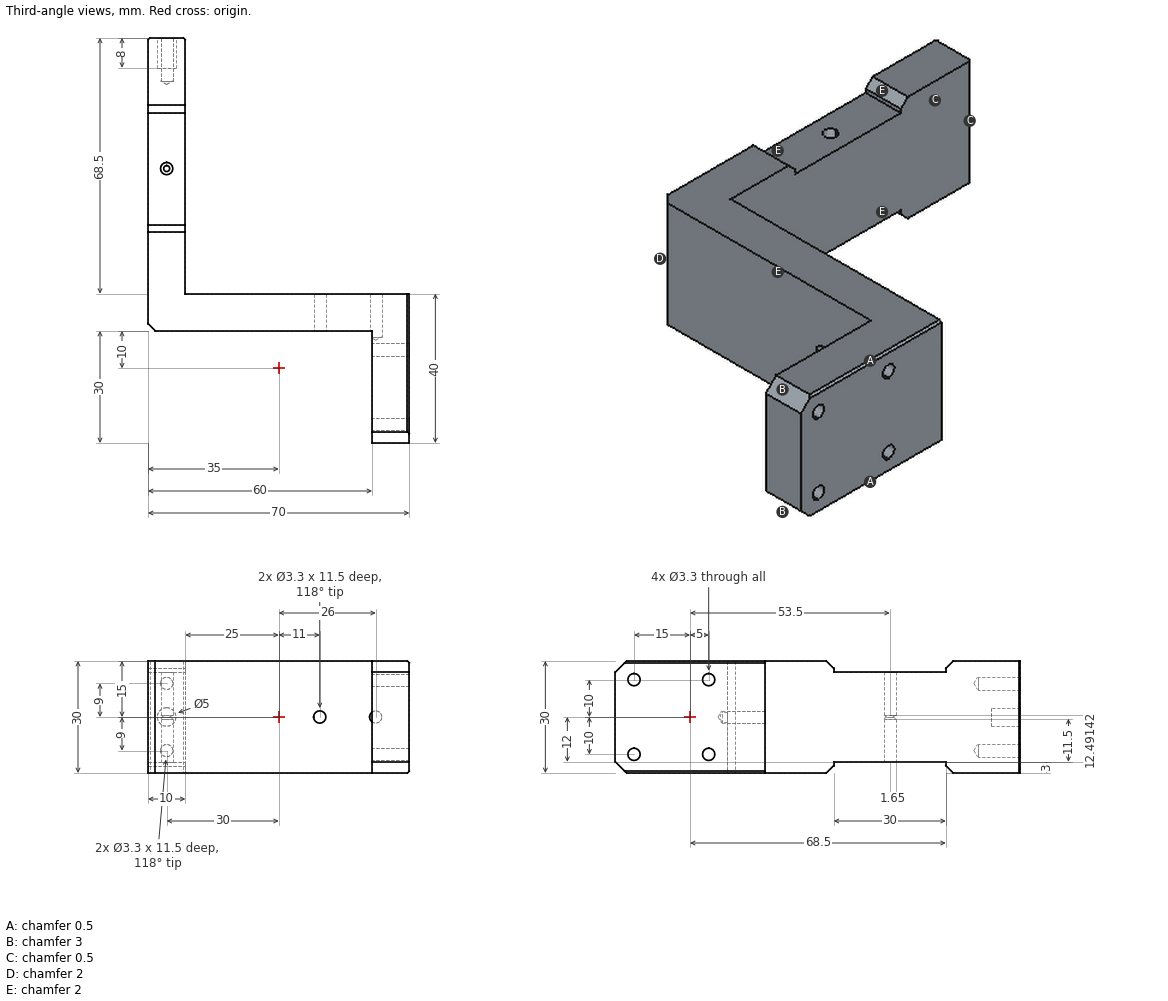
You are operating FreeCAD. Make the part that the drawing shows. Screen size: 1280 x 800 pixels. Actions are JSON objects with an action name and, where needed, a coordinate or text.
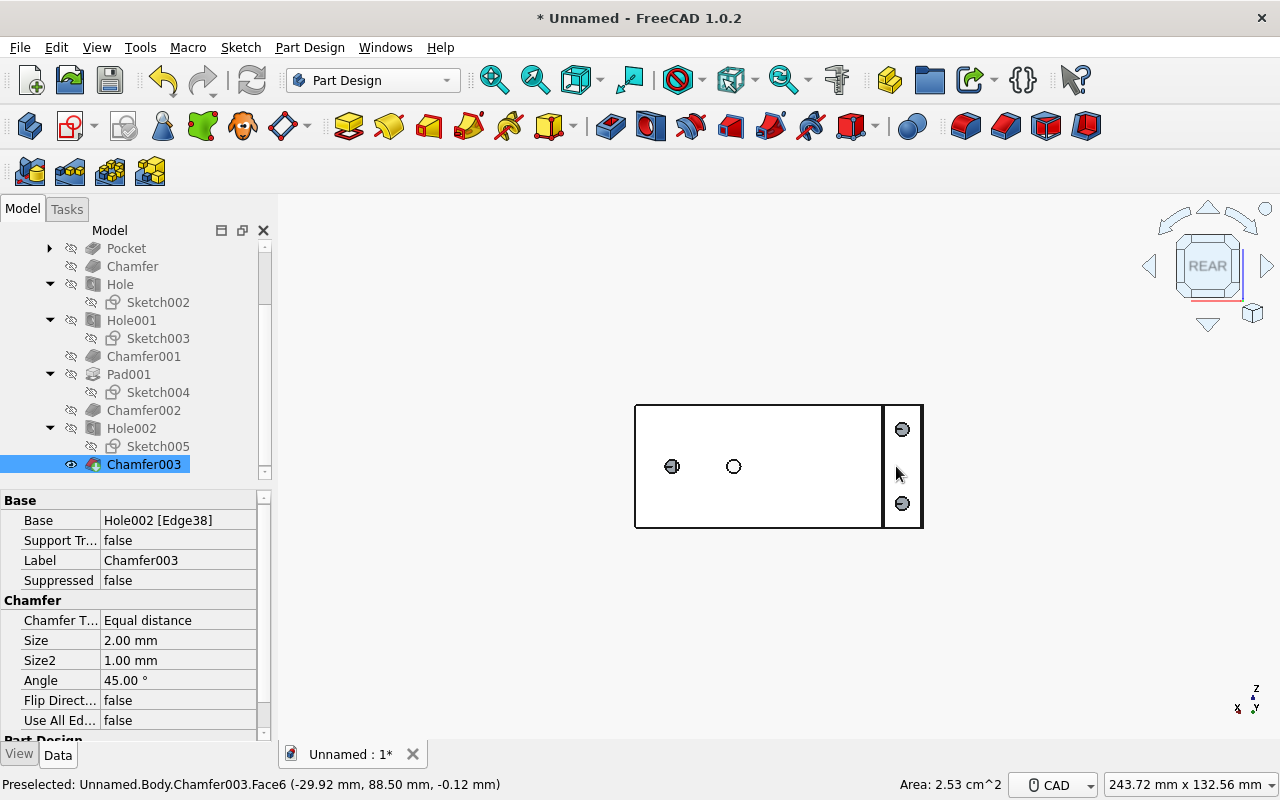
{"action": "left_click", "coordinate": [70, 126]}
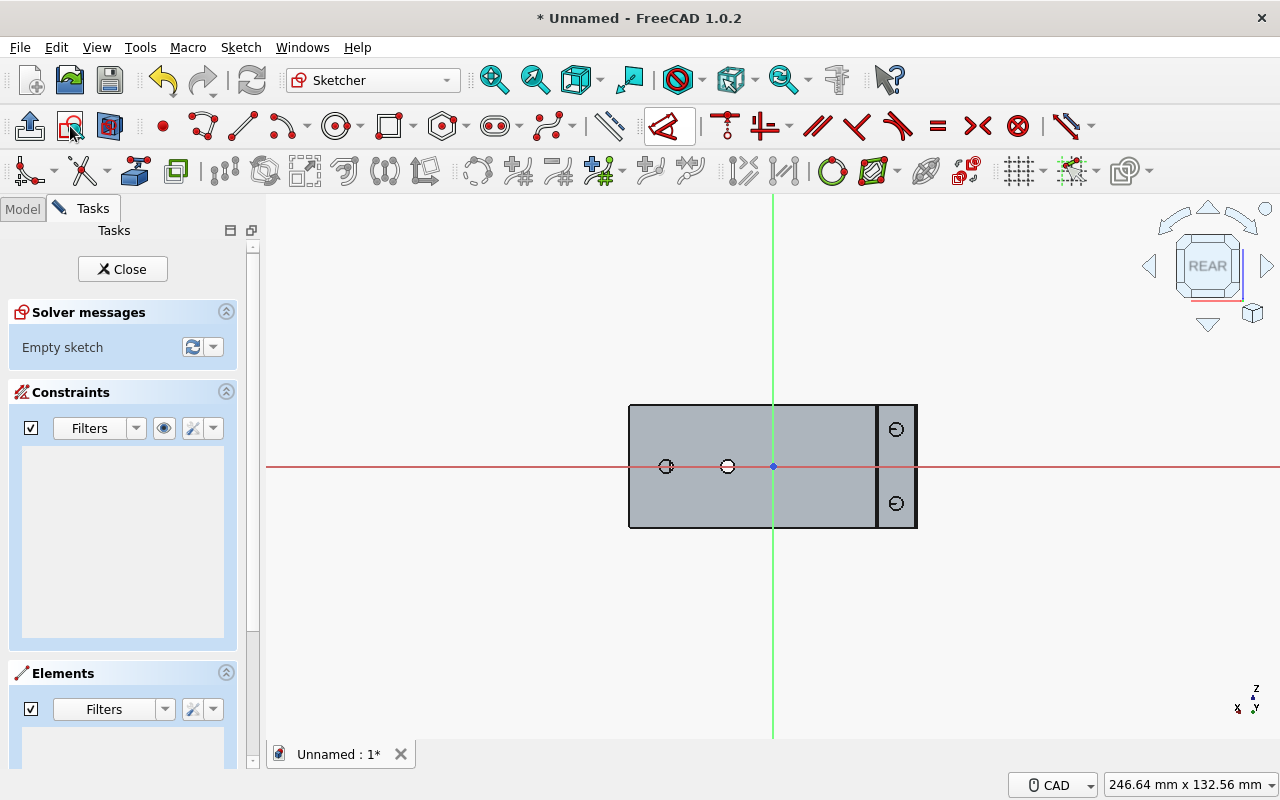
{"action": "scroll", "coordinate": [909, 467], "scroll_direction": "up", "scroll_amount": 14}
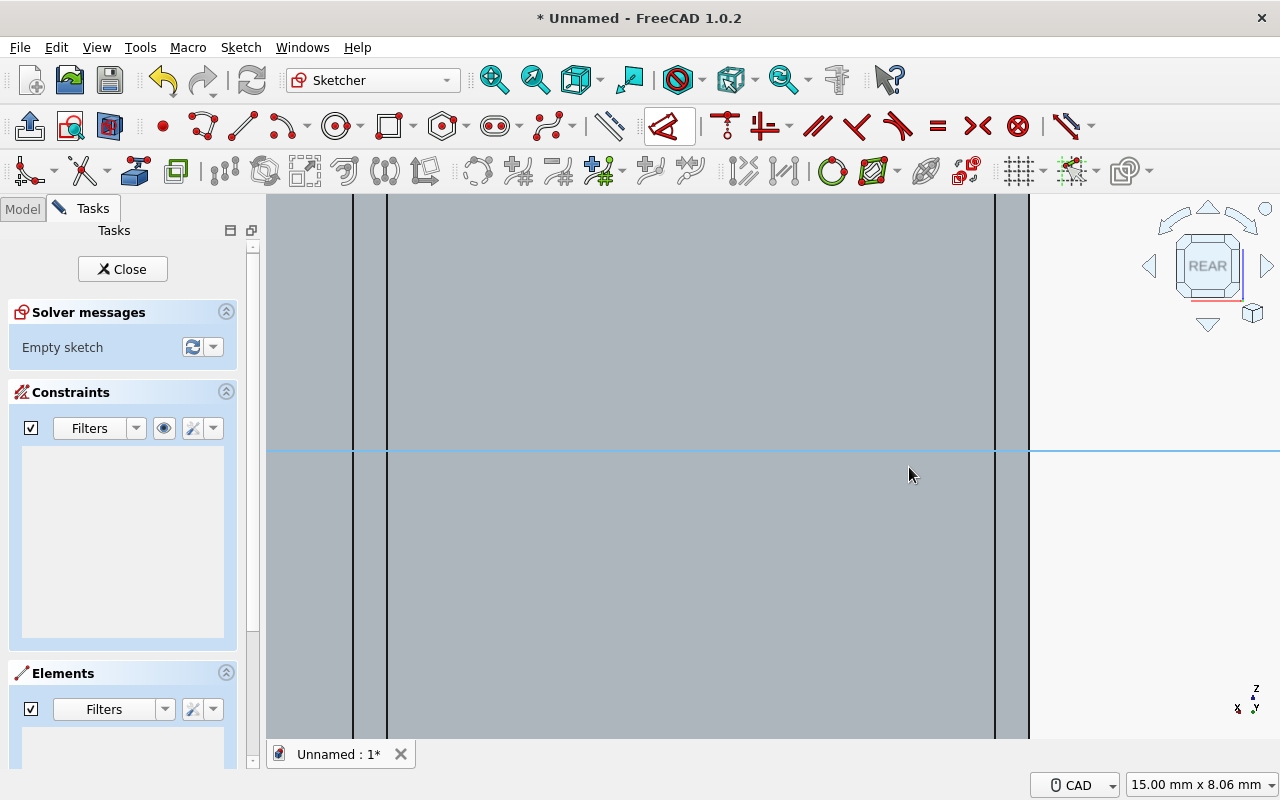
{"action": "left_click", "coordinate": [336, 126]}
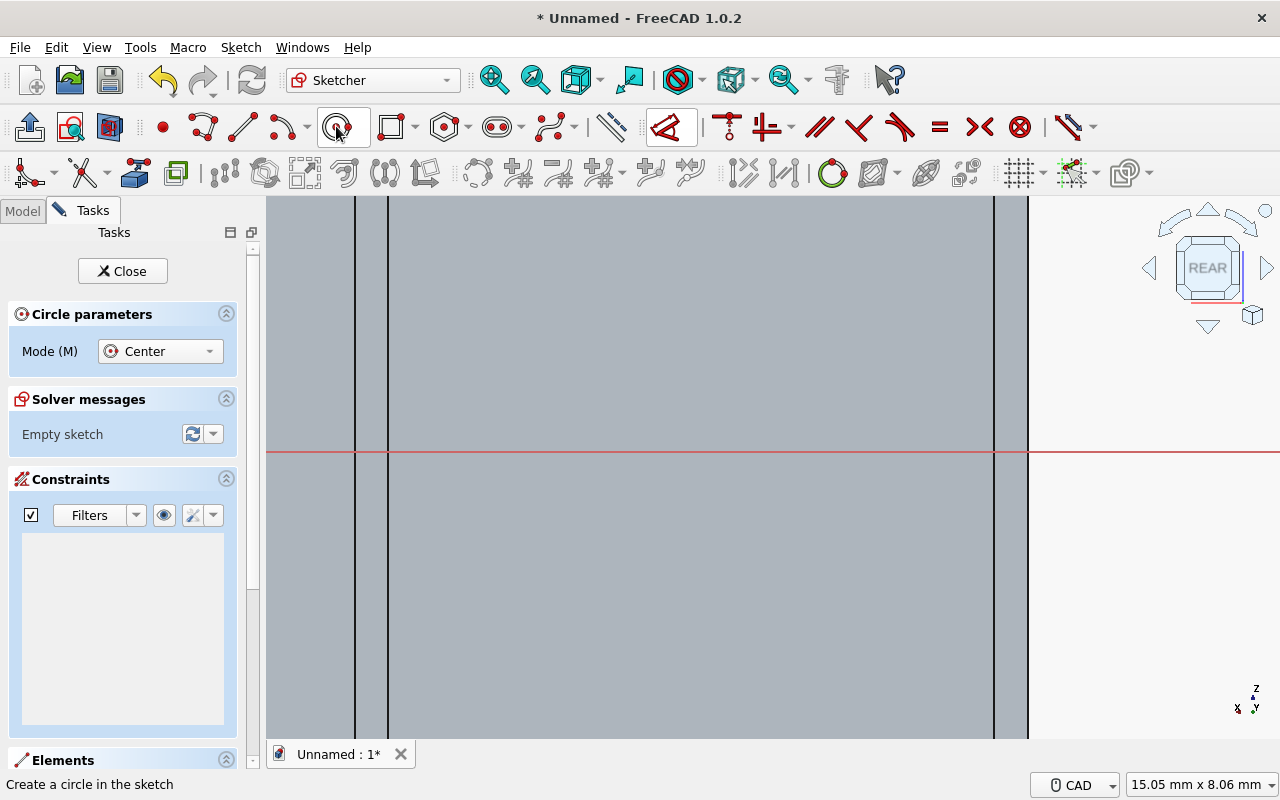
{"action": "left_click", "coordinate": [691, 452]}
{"action": "left_click", "coordinate": [810, 333]}
{"action": "key", "text": "Escape"}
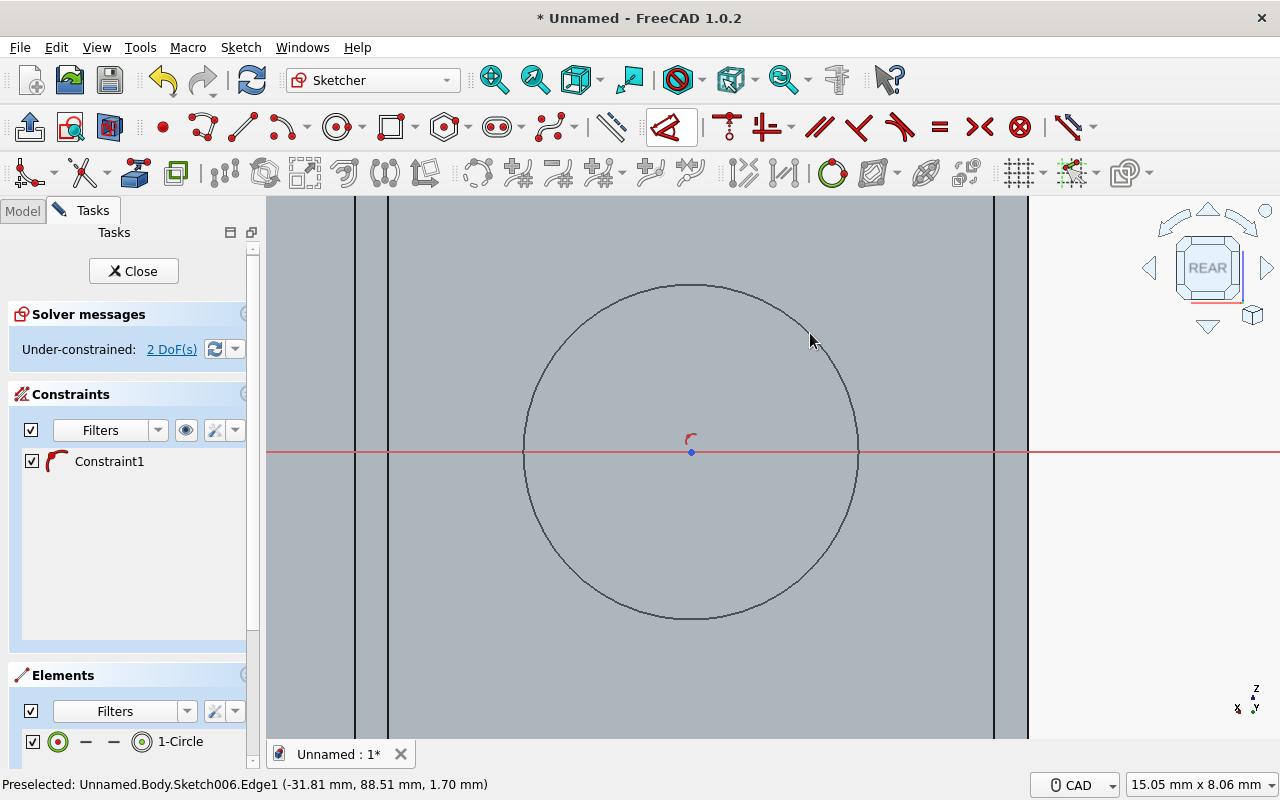
{"action": "left_click", "coordinate": [809, 333]}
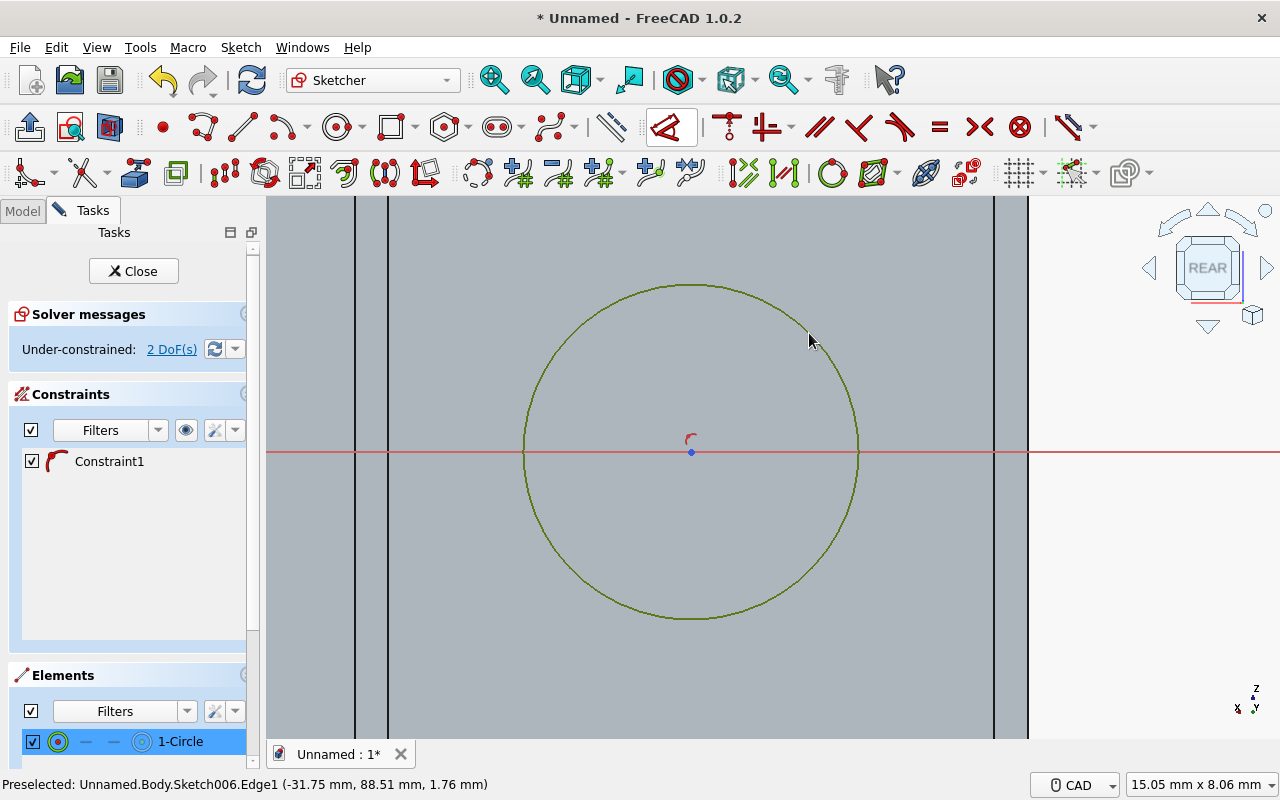
{"action": "left_click", "coordinate": [692, 128]}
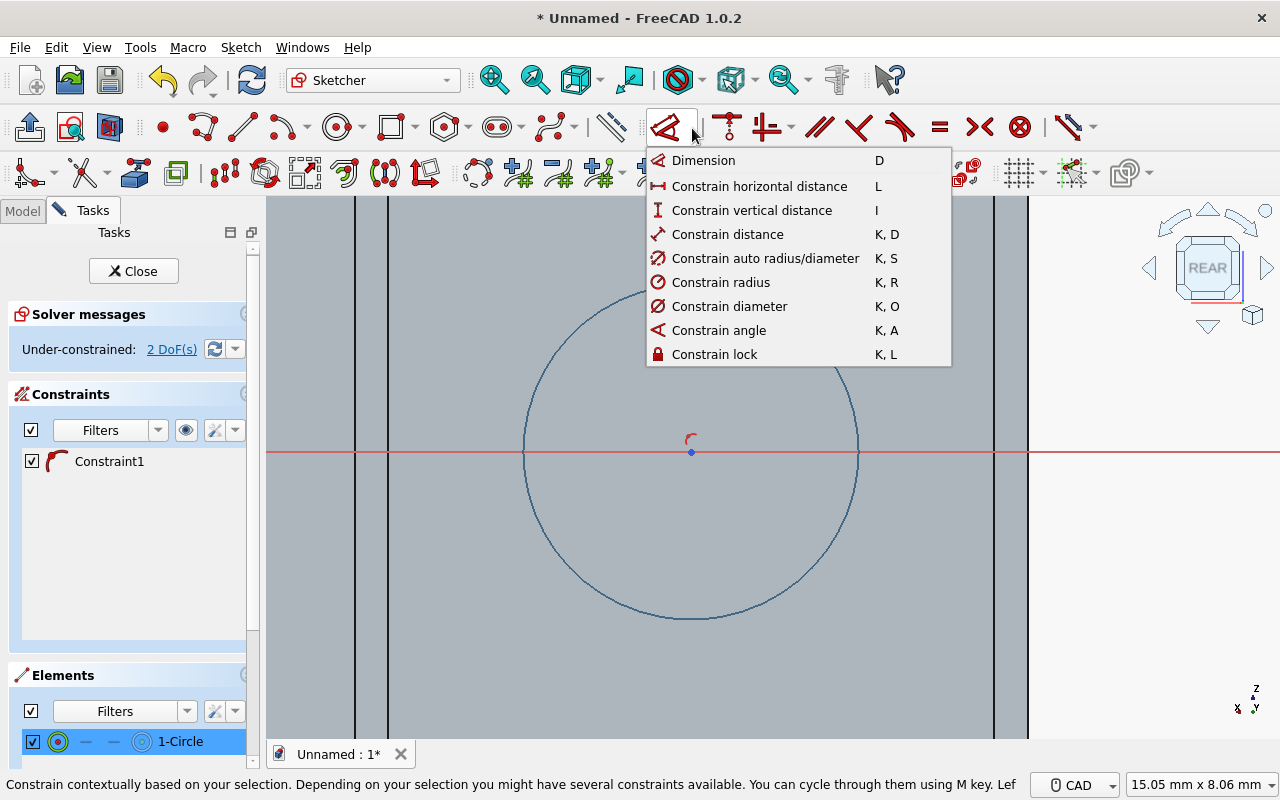
{"action": "left_click", "coordinate": [799, 306]}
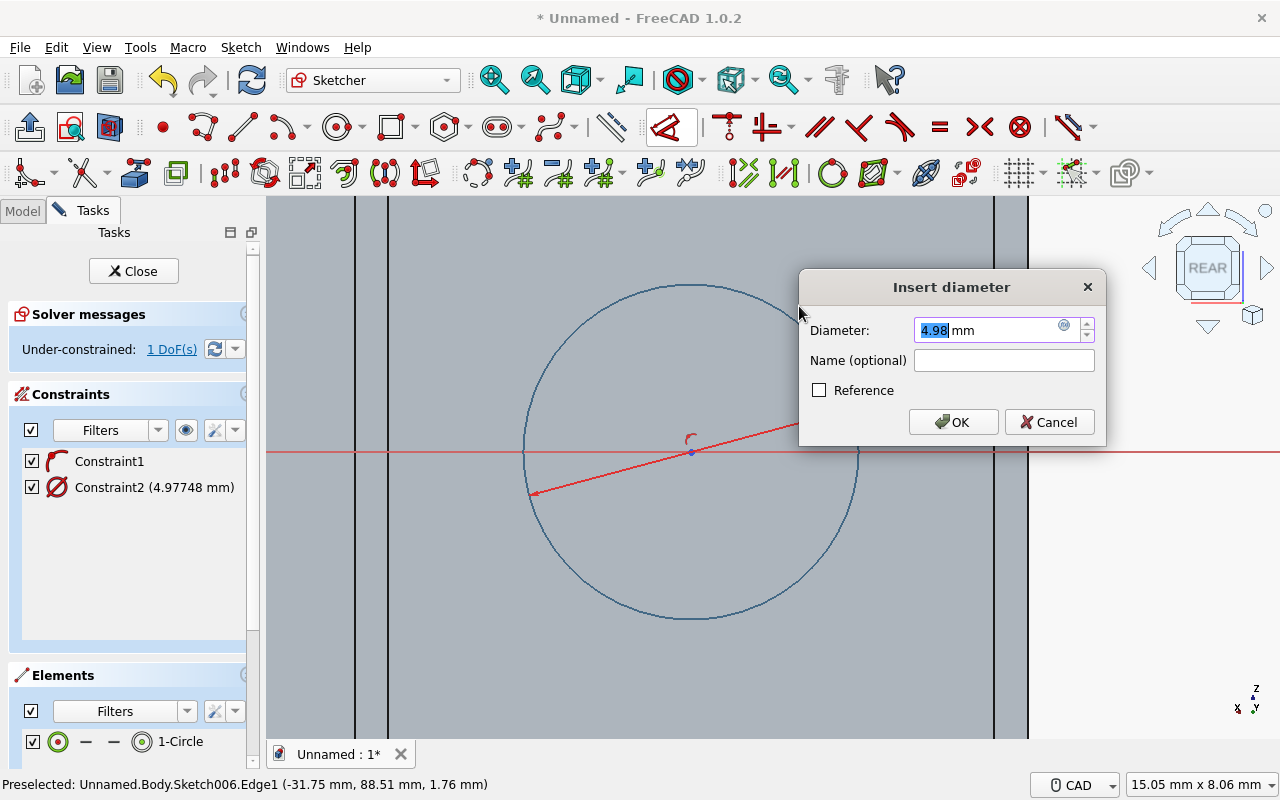
{"action": "type", "text": "5"}
{"action": "key", "text": "Return"}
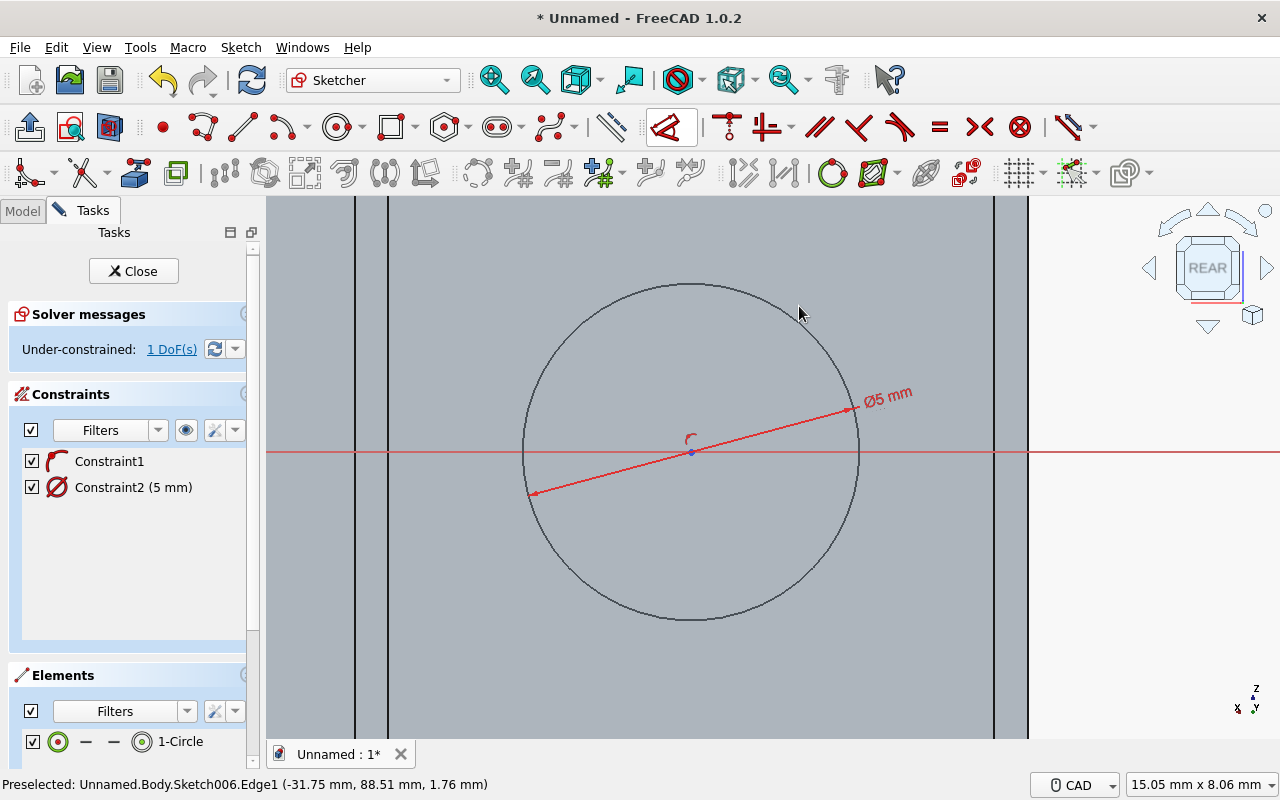
{"action": "left_click", "coordinate": [691, 452]}